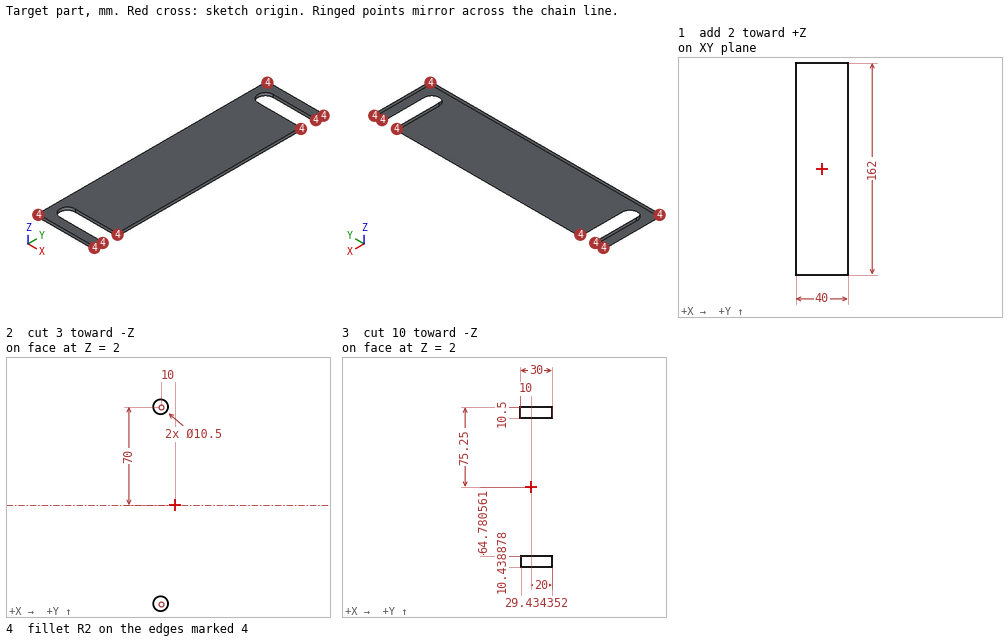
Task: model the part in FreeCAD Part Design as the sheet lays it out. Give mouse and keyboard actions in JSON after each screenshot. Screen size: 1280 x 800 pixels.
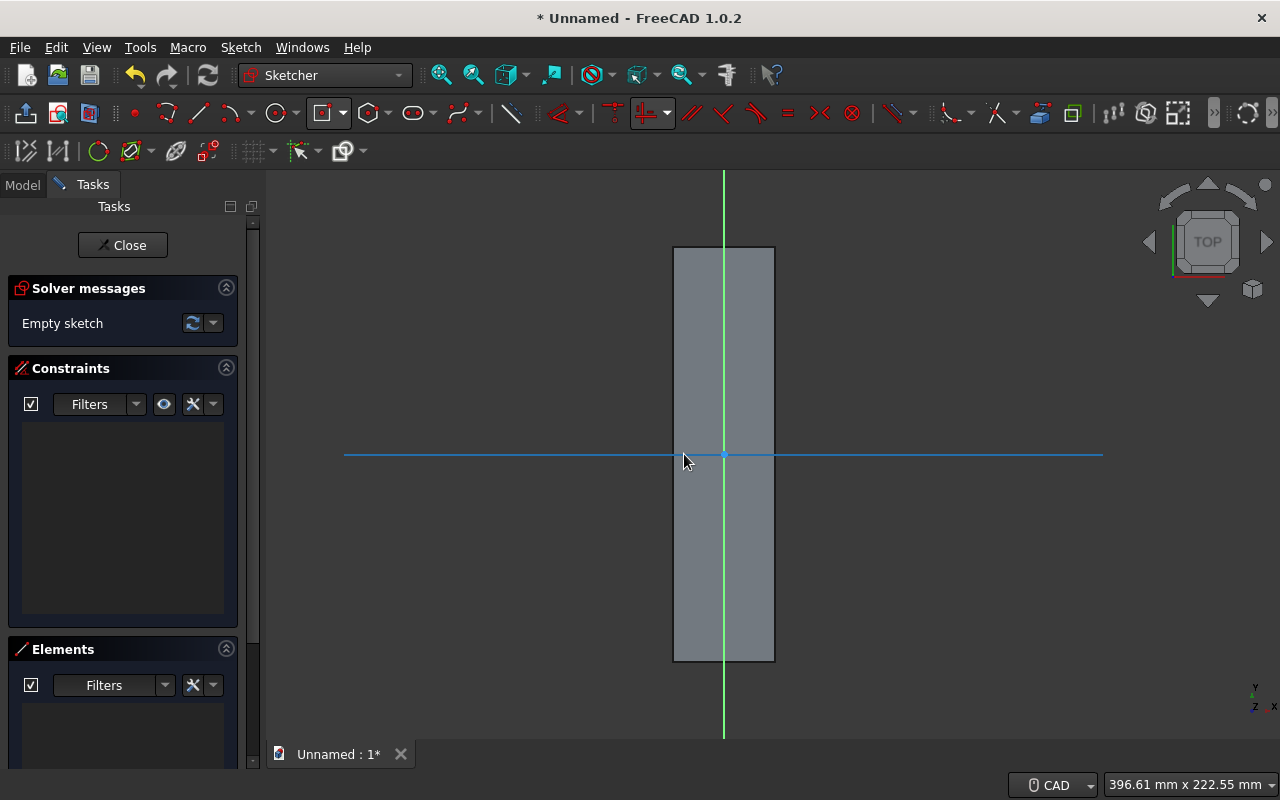
{"action": "left_click", "coordinate": [276, 114]}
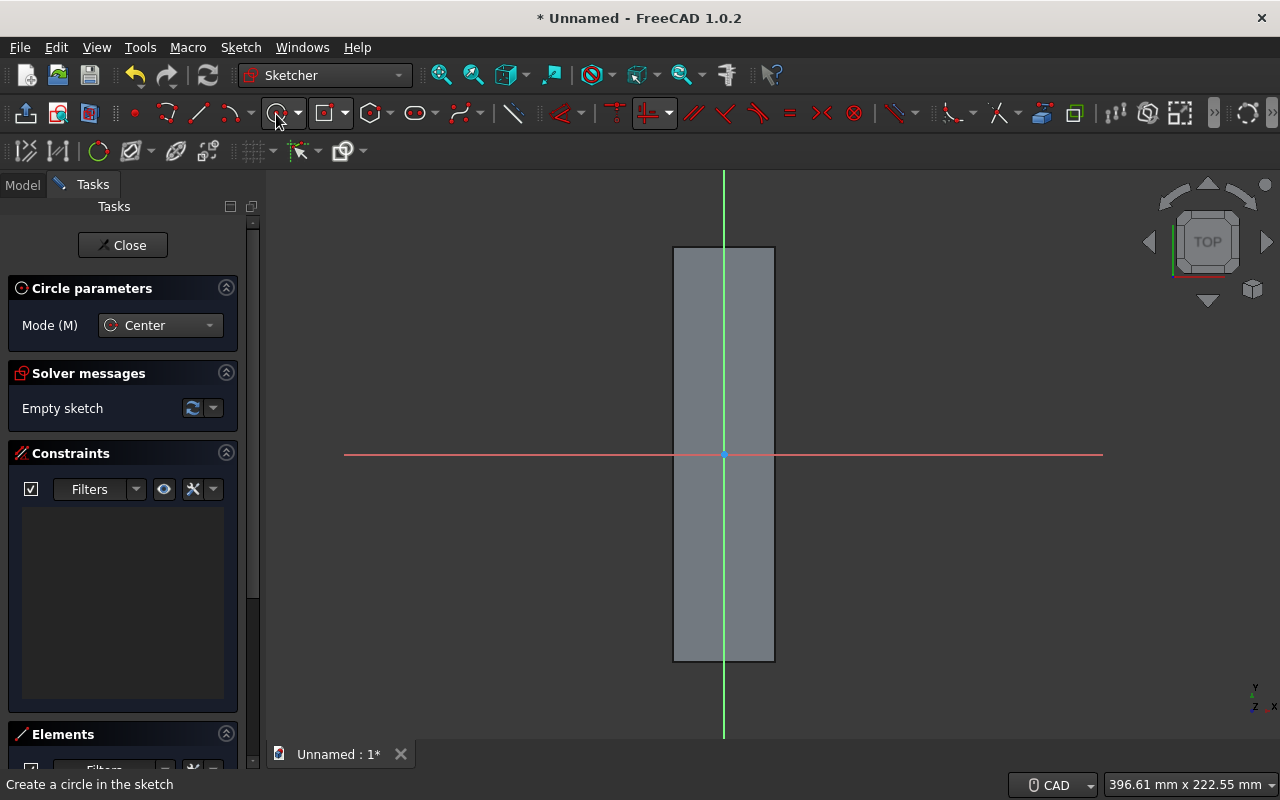
{"action": "scroll", "coordinate": [699, 276], "scroll_direction": "up", "scroll_amount": 3}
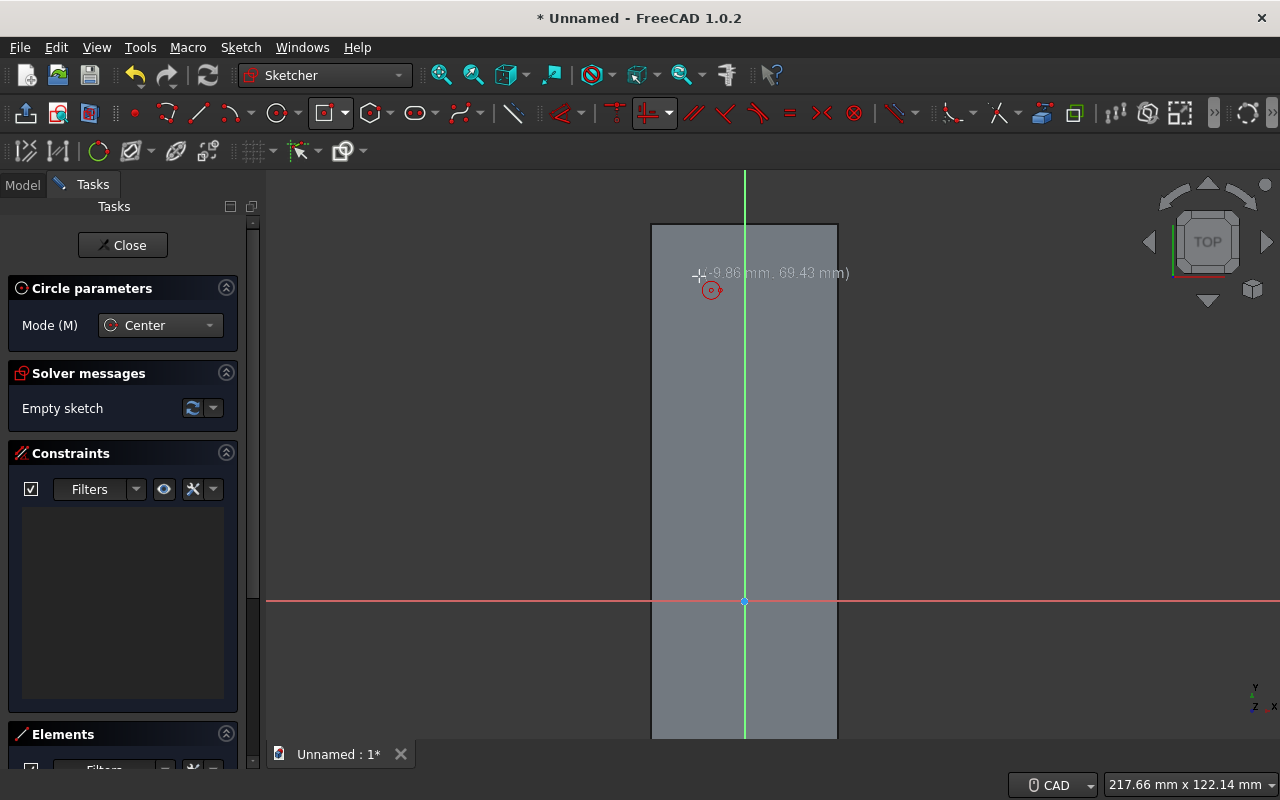
{"action": "left_click", "coordinate": [698, 275]}
{"action": "left_click", "coordinate": [715, 258]}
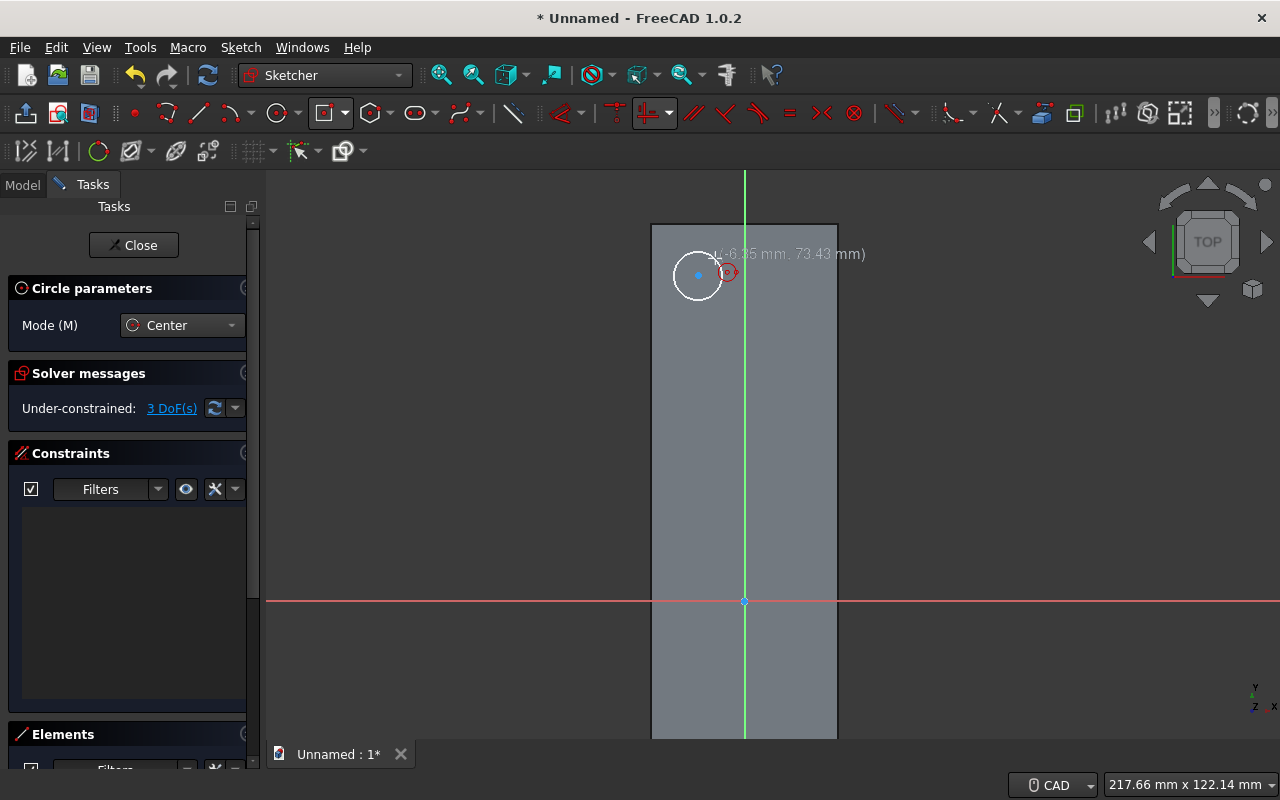
{"action": "scroll", "coordinate": [699, 276], "scroll_direction": "down", "scroll_amount": 3}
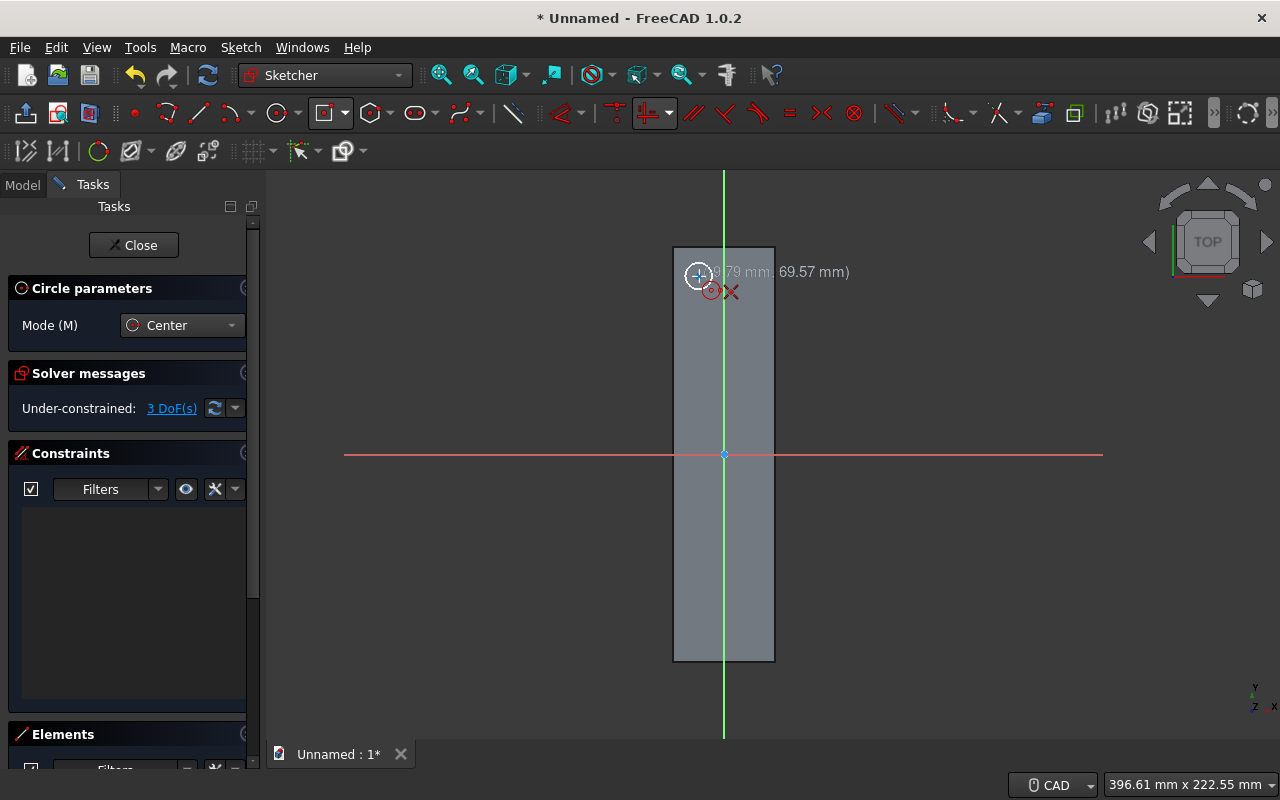
{"action": "scroll", "coordinate": [699, 633], "scroll_direction": "up", "scroll_amount": 3}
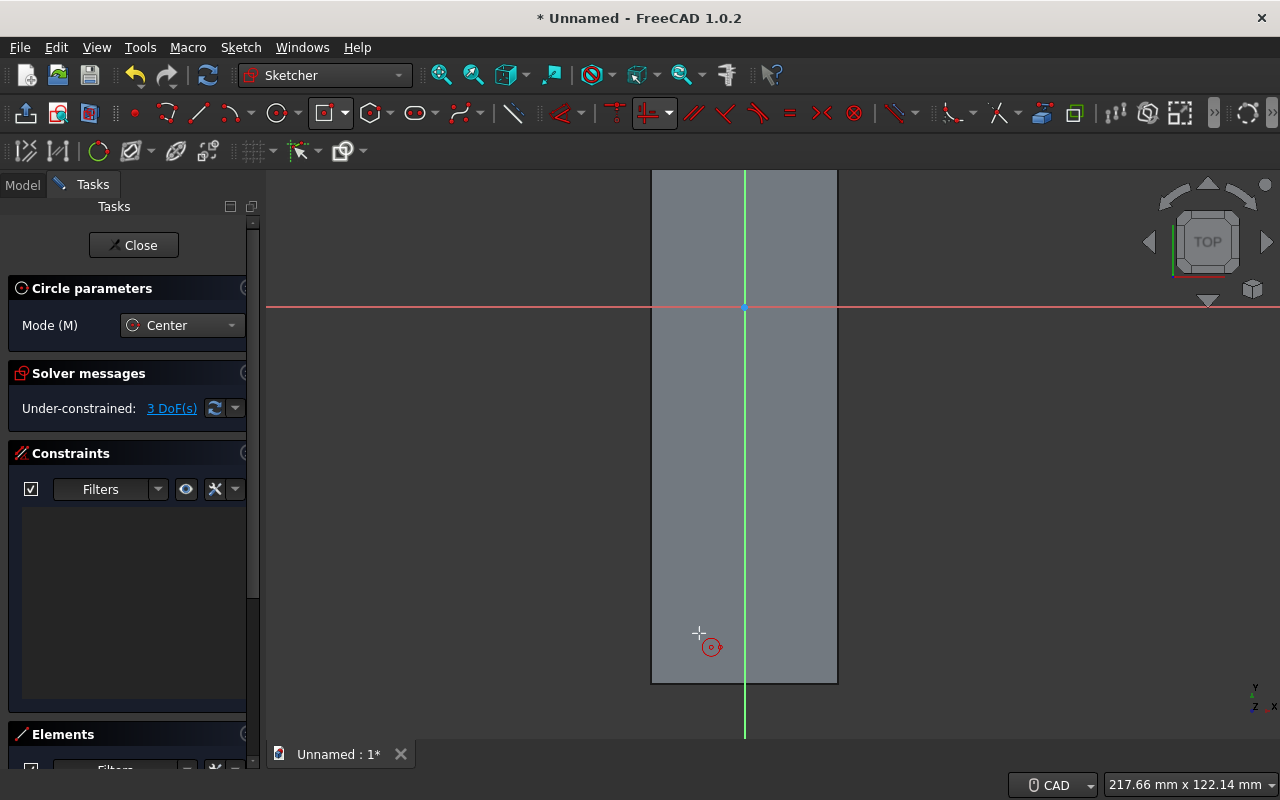
{"action": "left_click", "coordinate": [698, 633]}
{"action": "left_click", "coordinate": [715, 616]}
{"action": "key", "text": "Escape"}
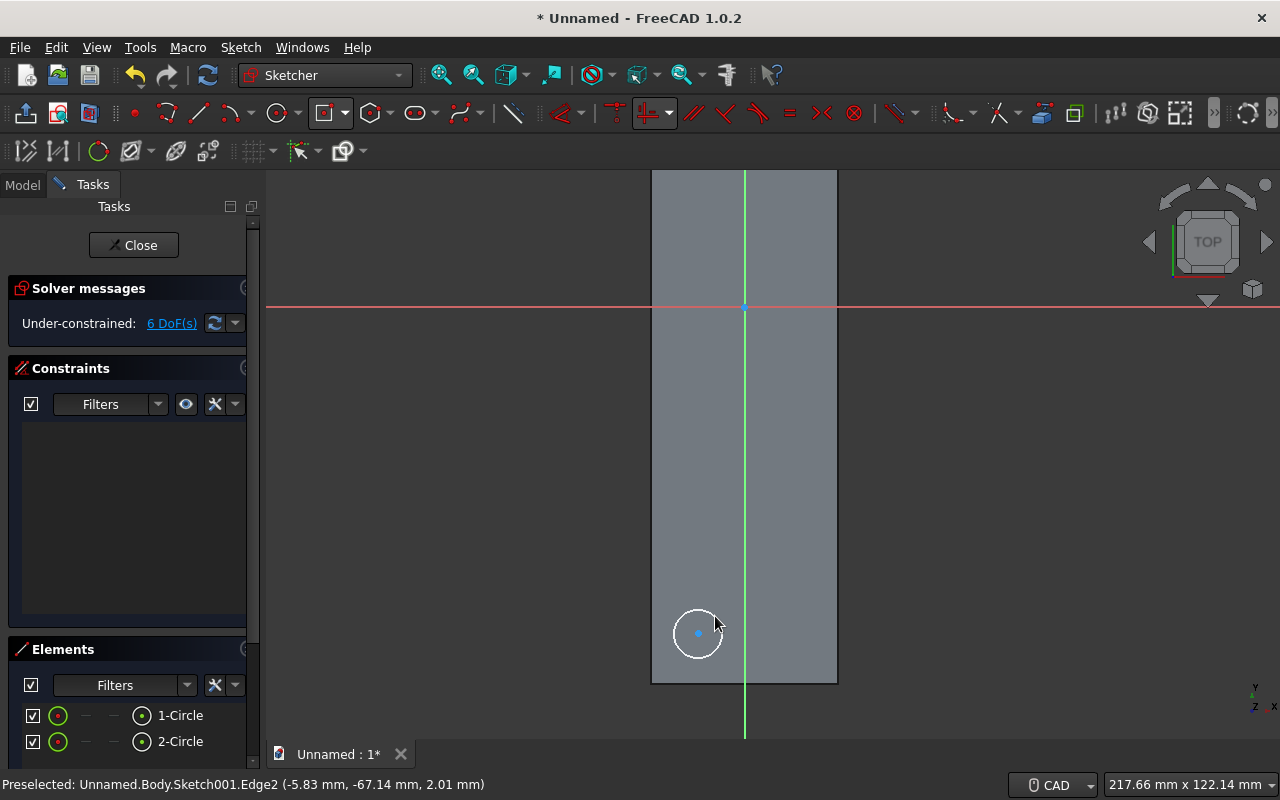
{"action": "scroll", "coordinate": [699, 634], "scroll_direction": "down", "scroll_amount": 3}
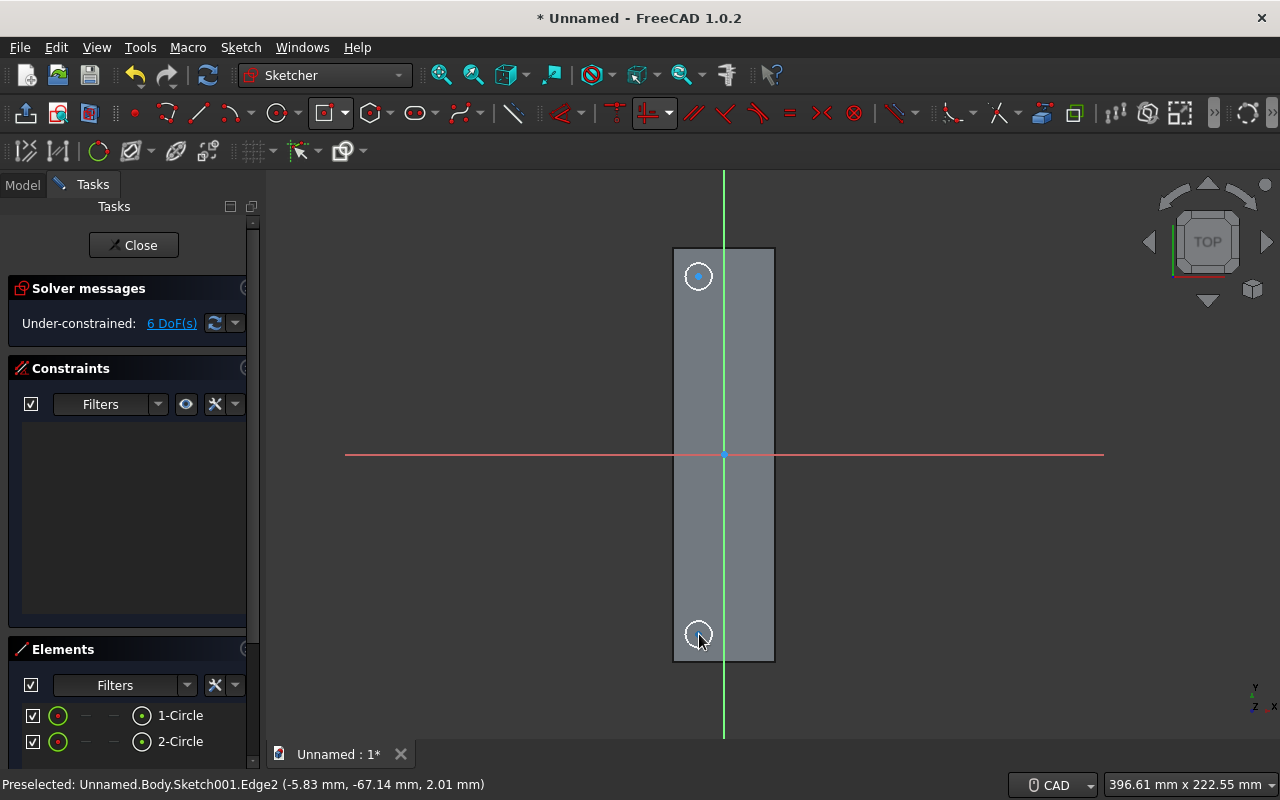
{"action": "left_click", "coordinate": [708, 267]}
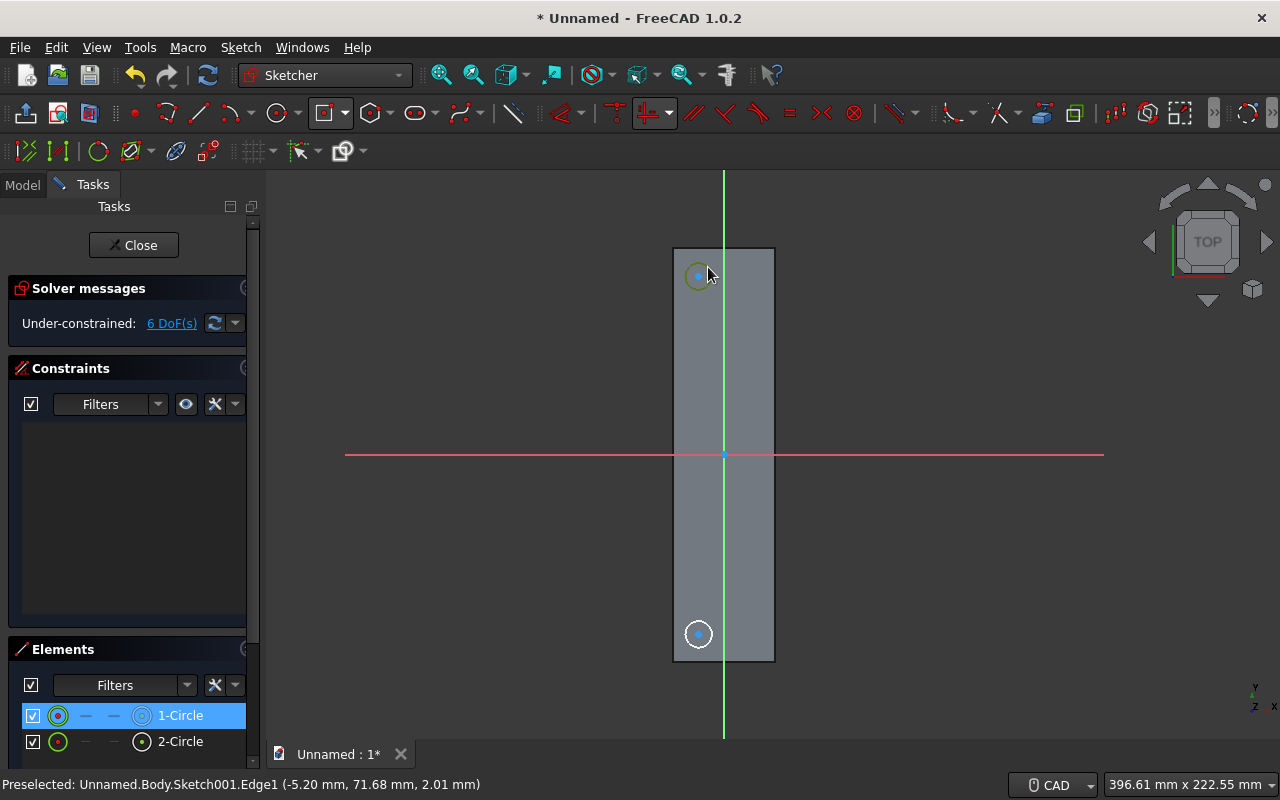
{"action": "left_click", "coordinate": [708, 625]}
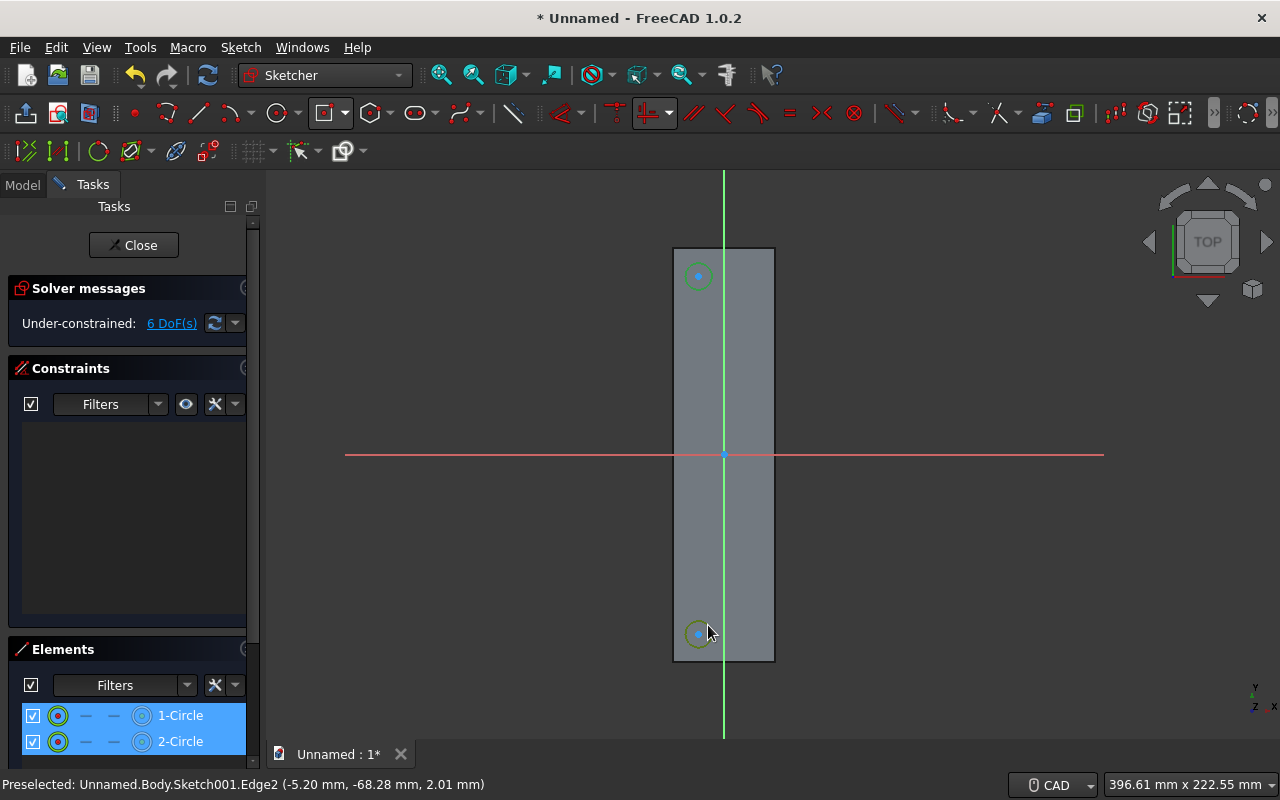
{"action": "left_click", "coordinate": [790, 114]}